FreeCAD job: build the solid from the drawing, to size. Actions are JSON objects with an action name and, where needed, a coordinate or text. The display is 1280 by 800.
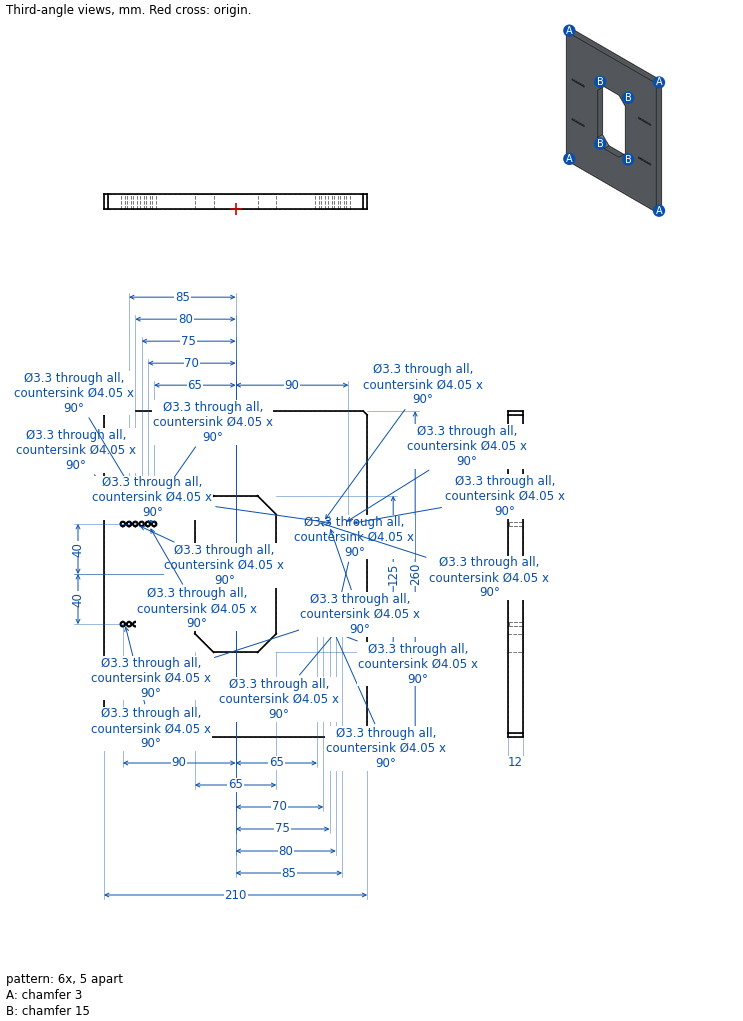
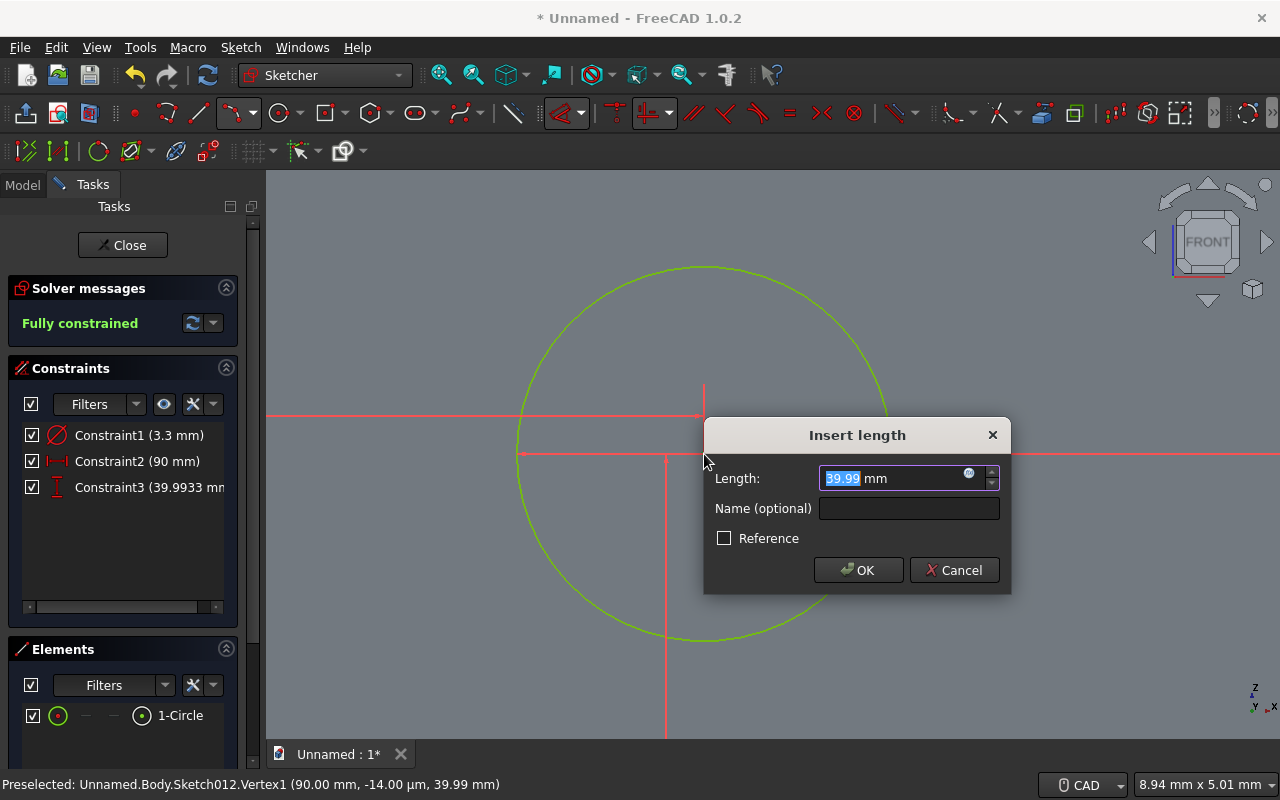
{"action": "type", "text": "40"}
{"action": "key", "text": "Return"}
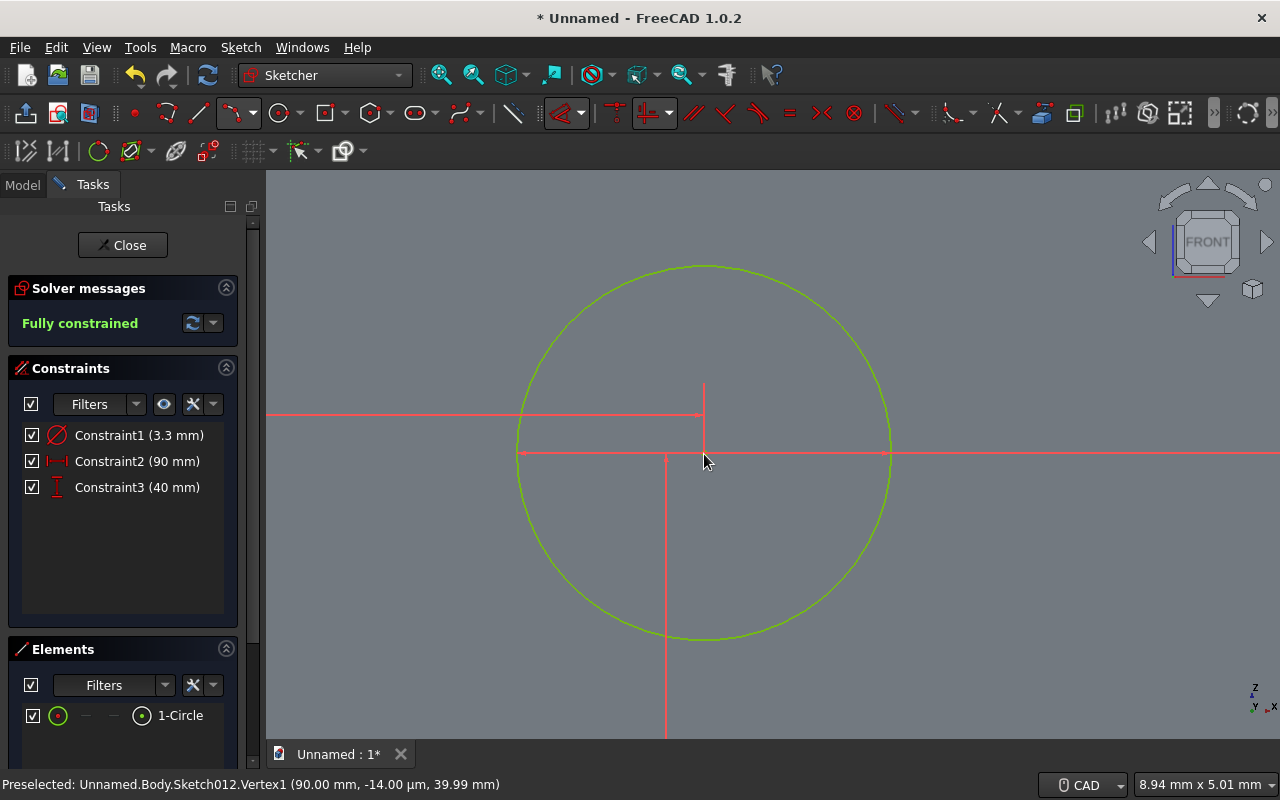
{"action": "left_click", "coordinate": [123, 245]}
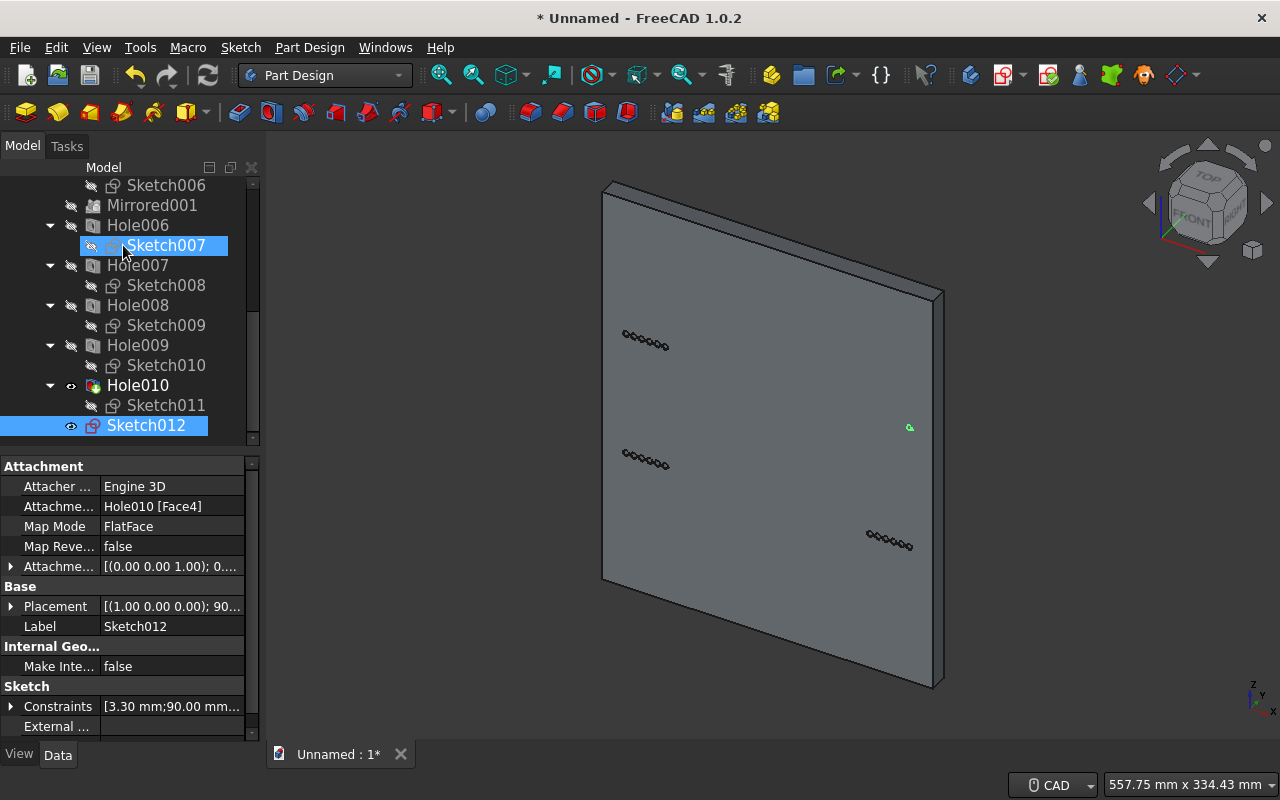
{"action": "left_click", "coordinate": [272, 112]}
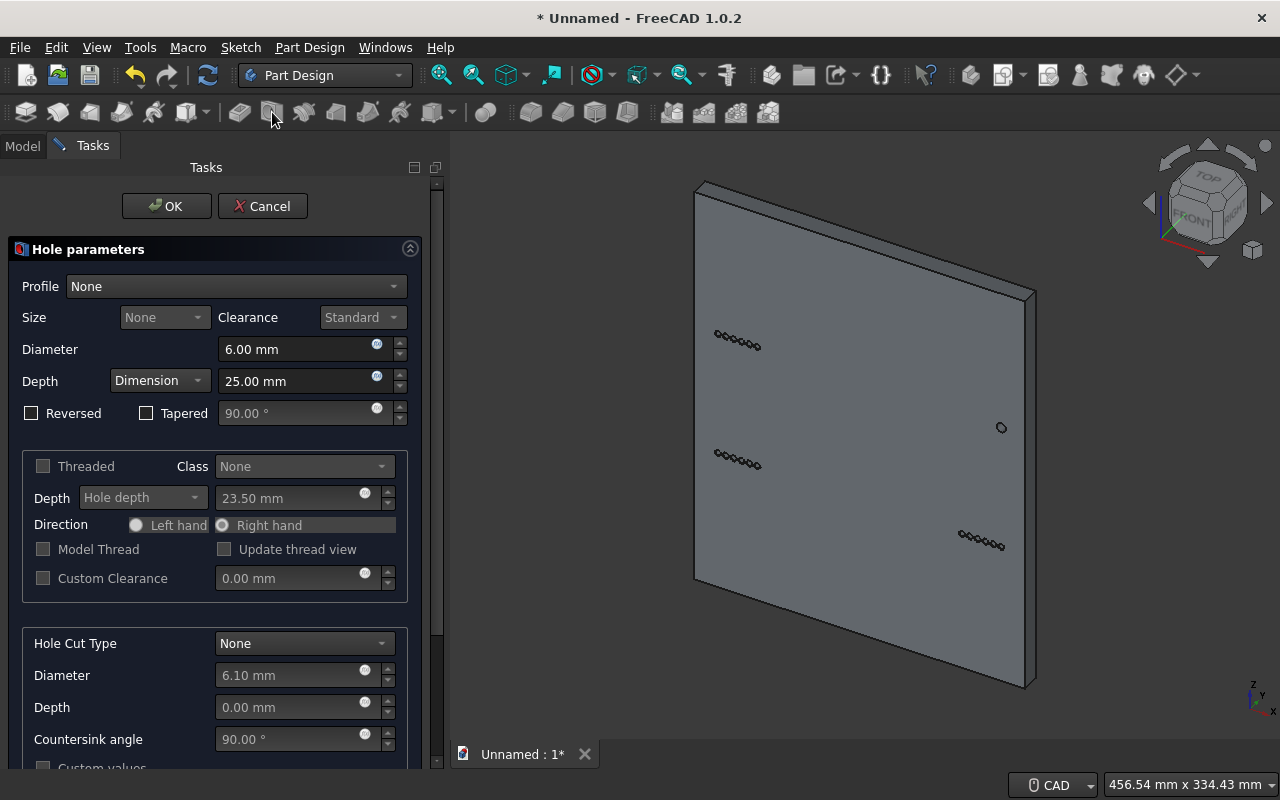
{"action": "triple_click", "coordinate": [305, 349]}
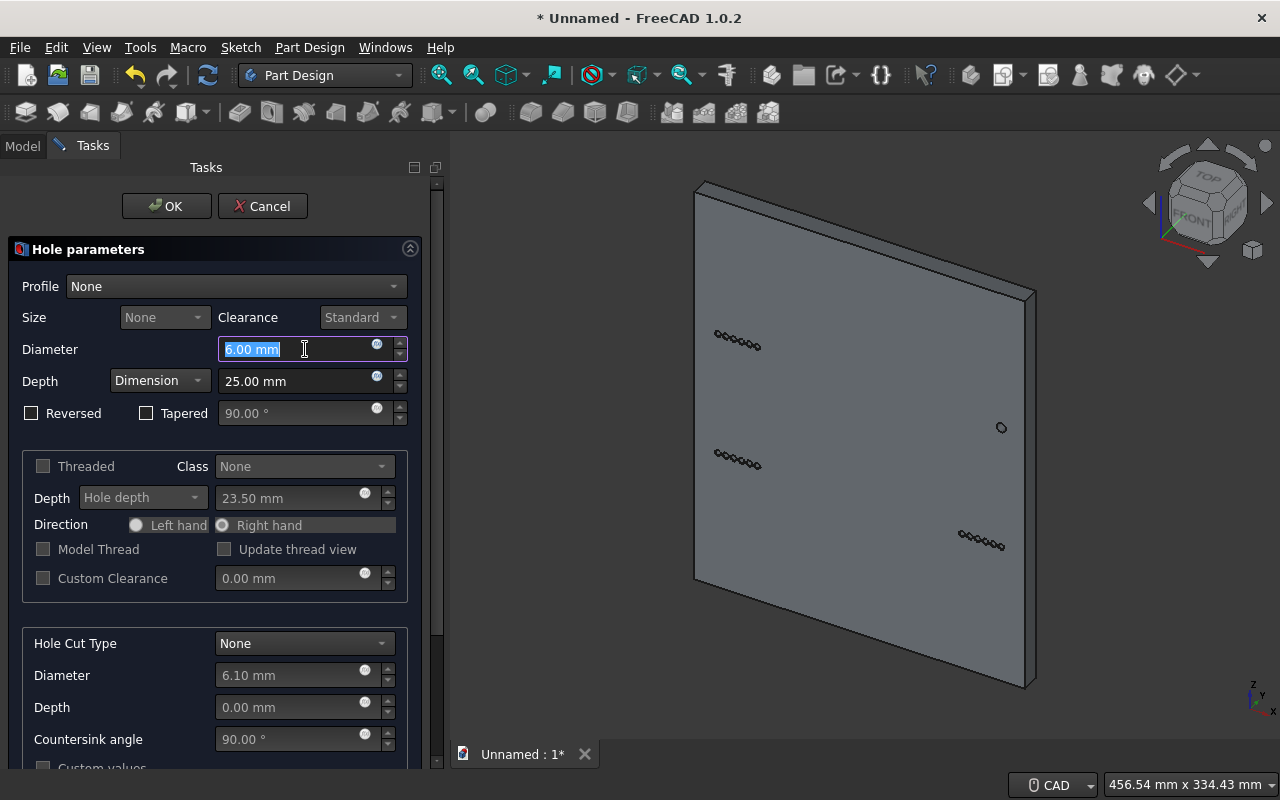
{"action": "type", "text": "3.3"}
{"action": "key", "text": "Tab"}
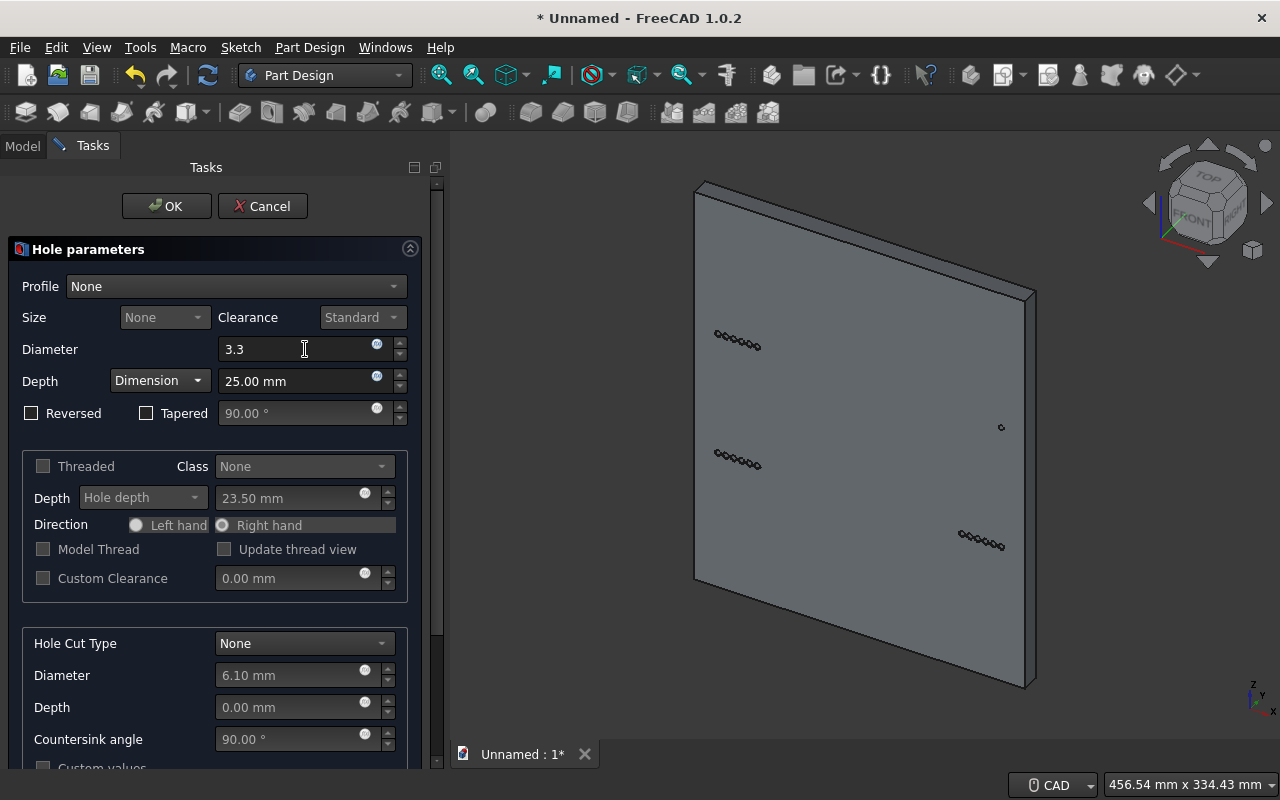
{"action": "left_click", "coordinate": [161, 380]}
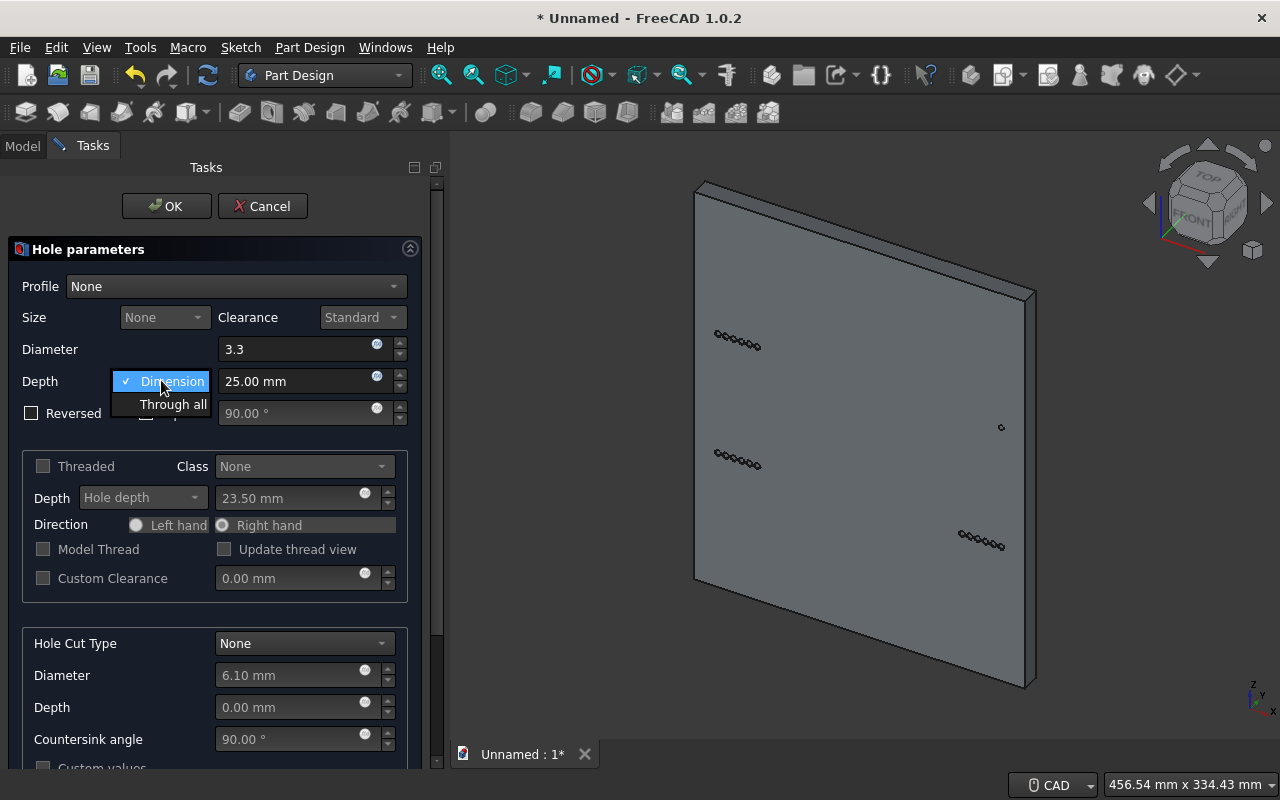
{"action": "left_click", "coordinate": [160, 404]}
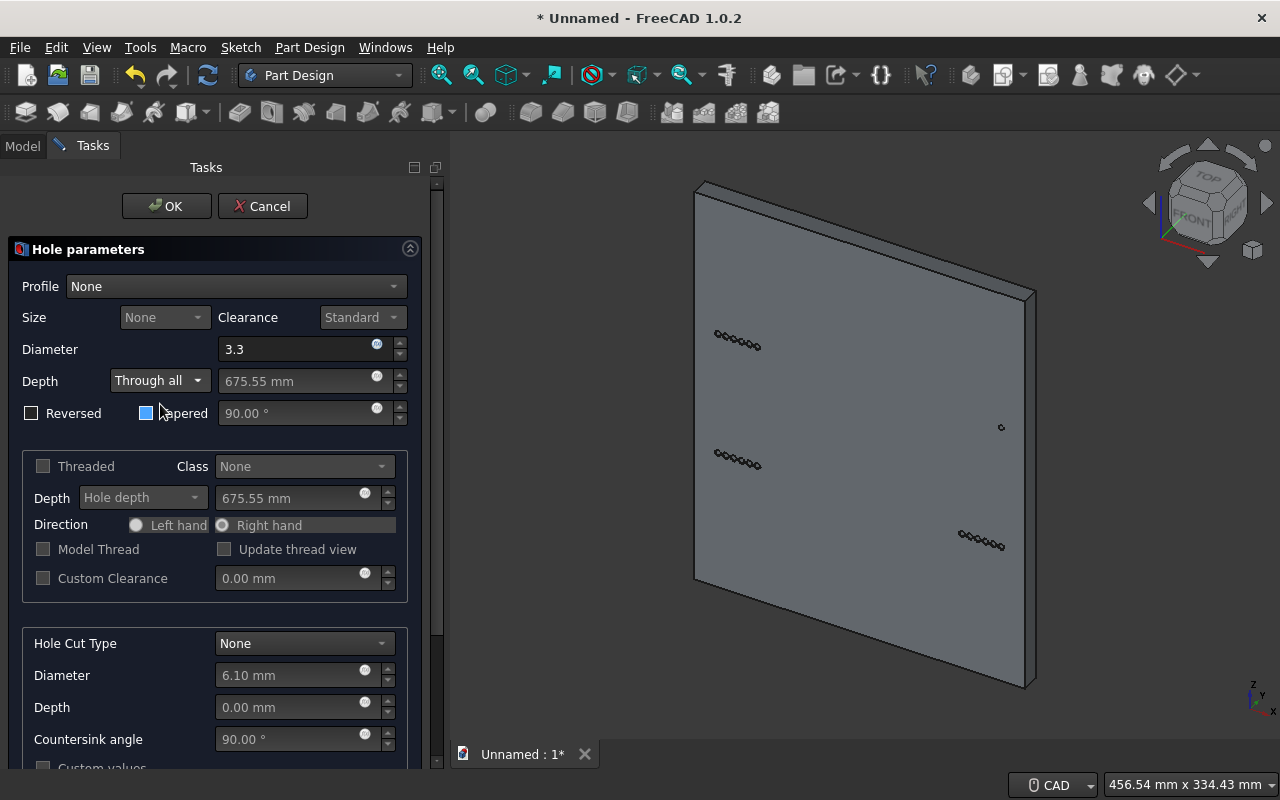
{"action": "left_click", "coordinate": [306, 644]}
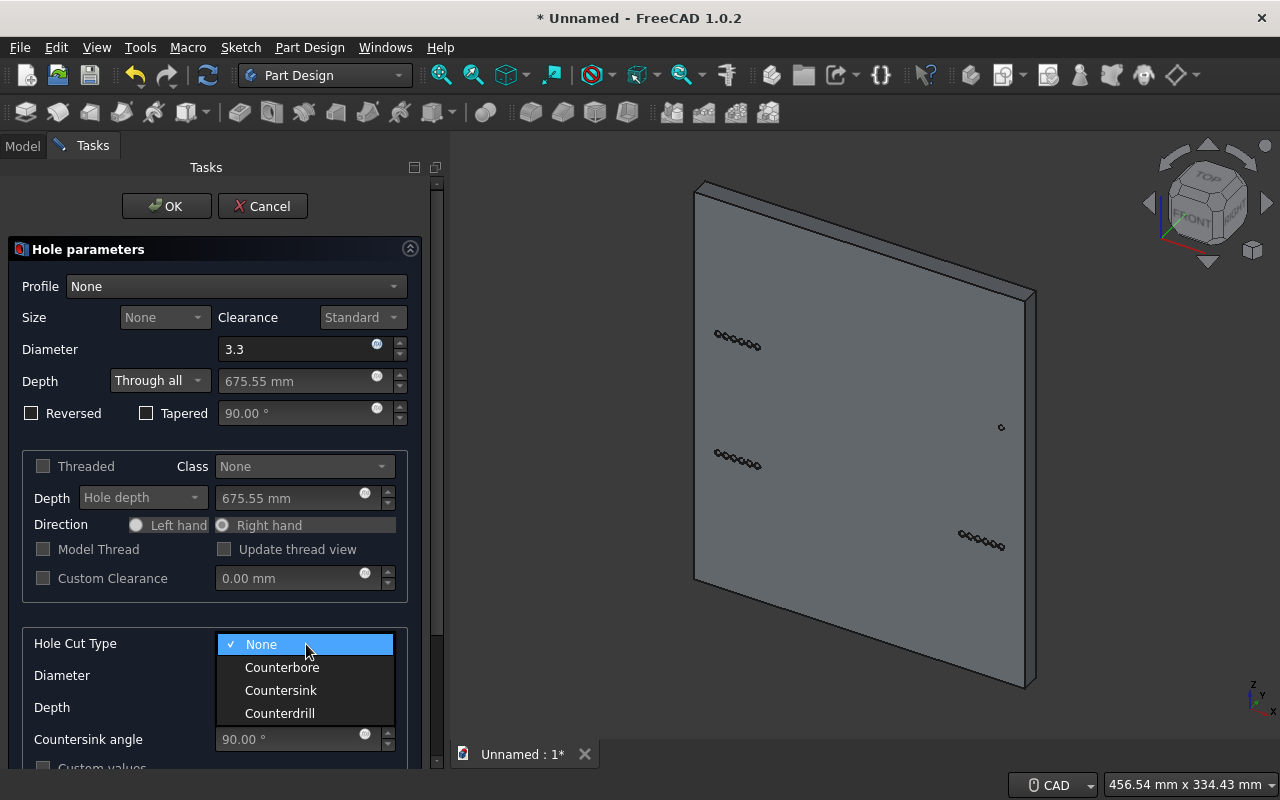
{"action": "left_click", "coordinate": [304, 690]}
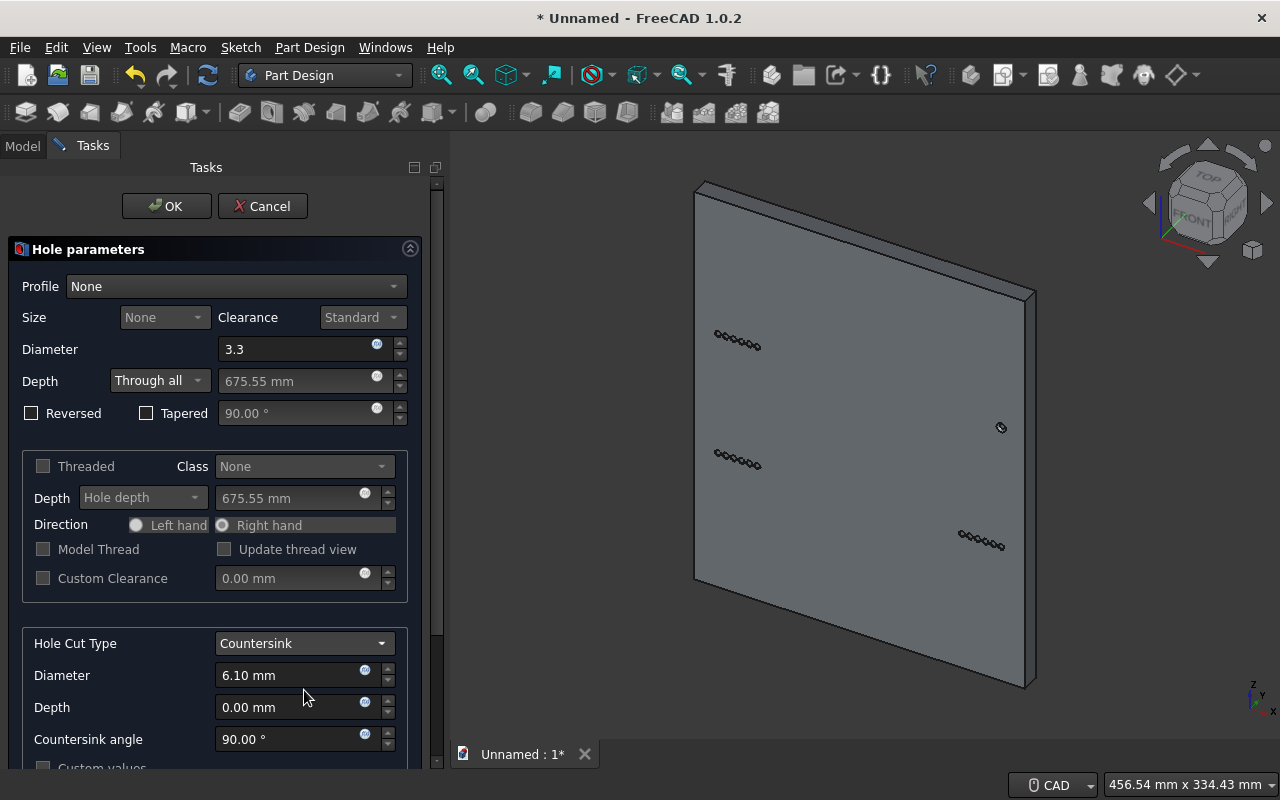
{"action": "triple_click", "coordinate": [298, 675]}